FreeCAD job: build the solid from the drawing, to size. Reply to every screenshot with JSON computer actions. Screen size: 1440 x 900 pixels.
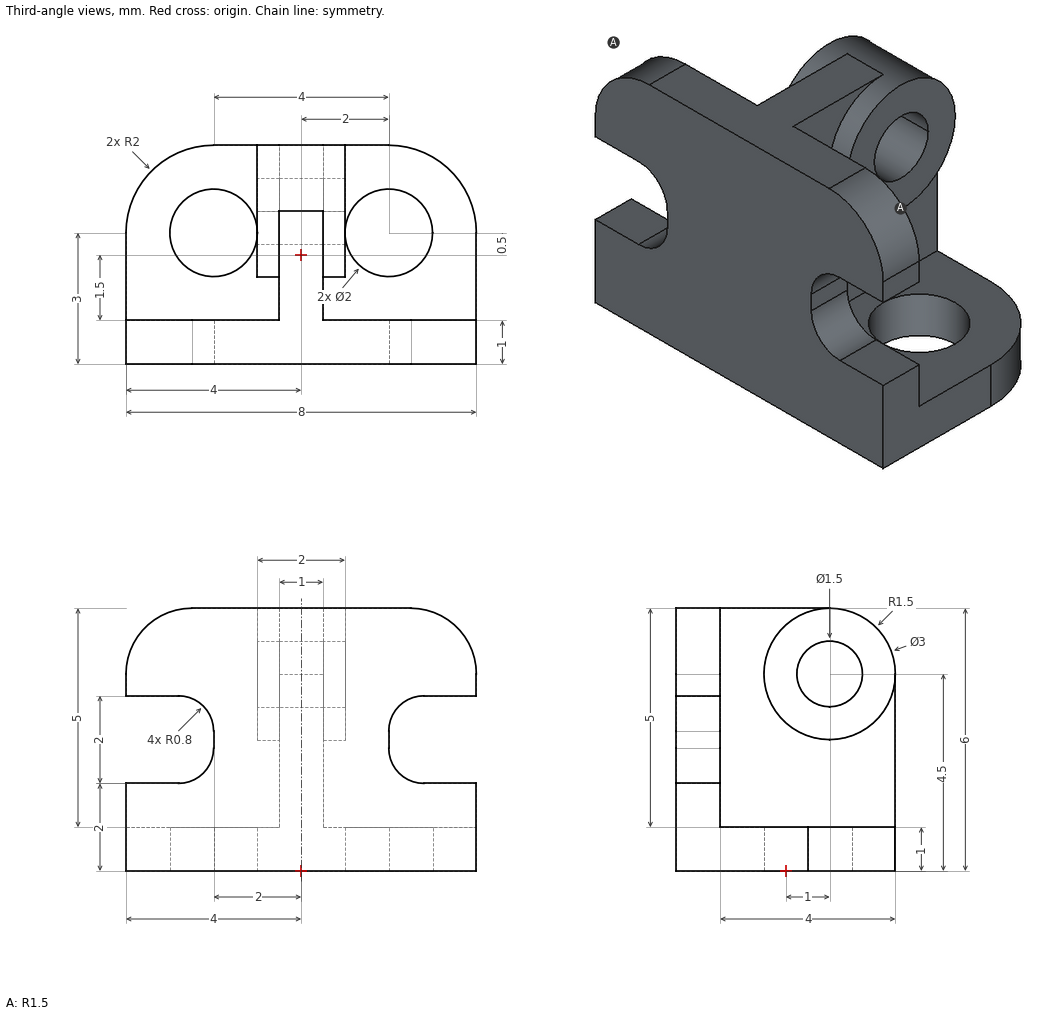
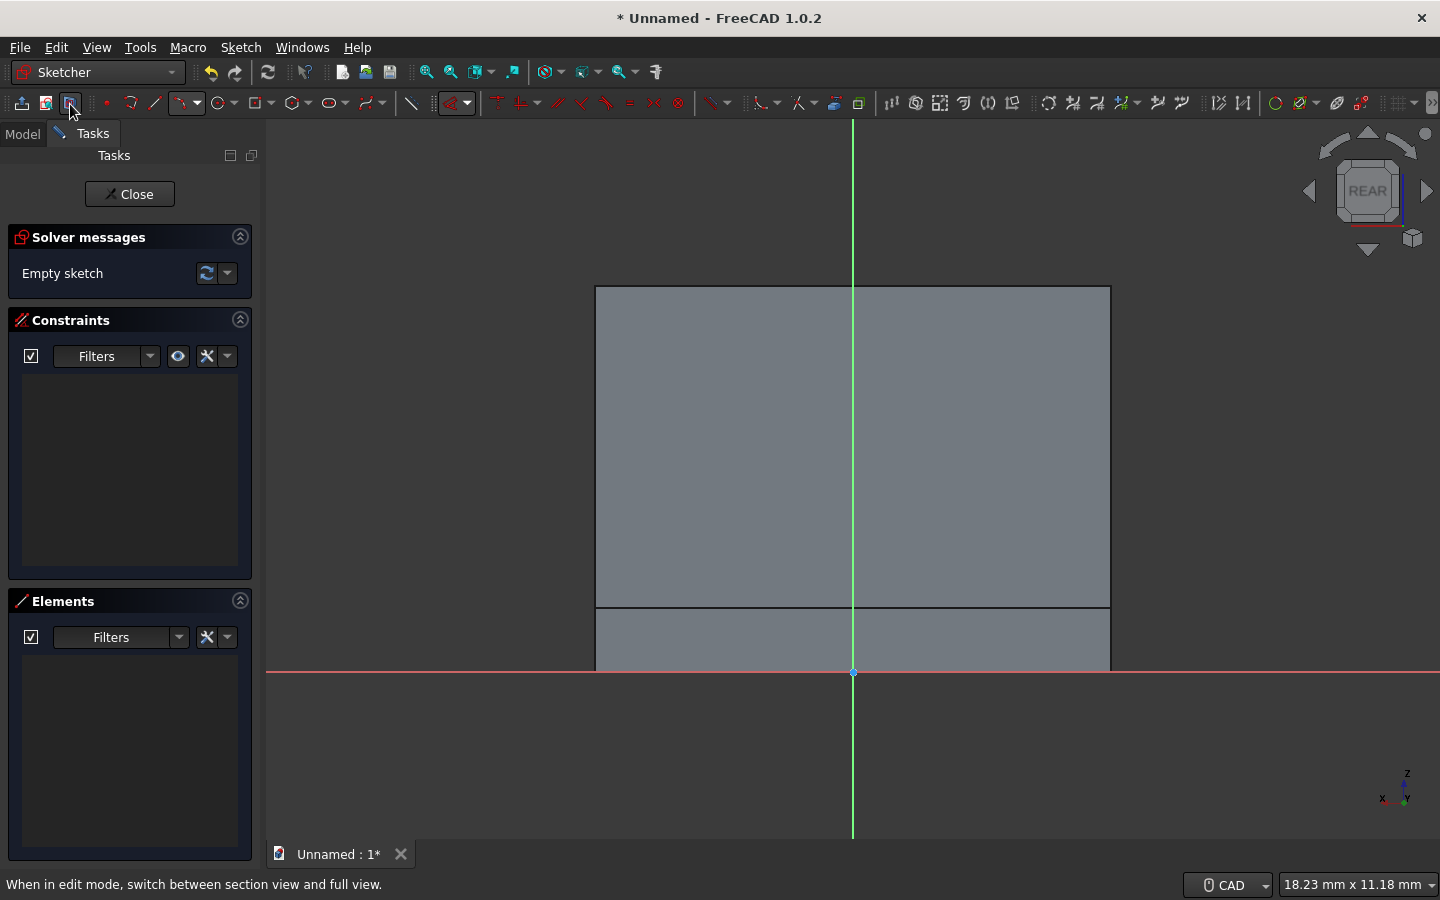
{"action": "left_click", "coordinate": [132, 104]}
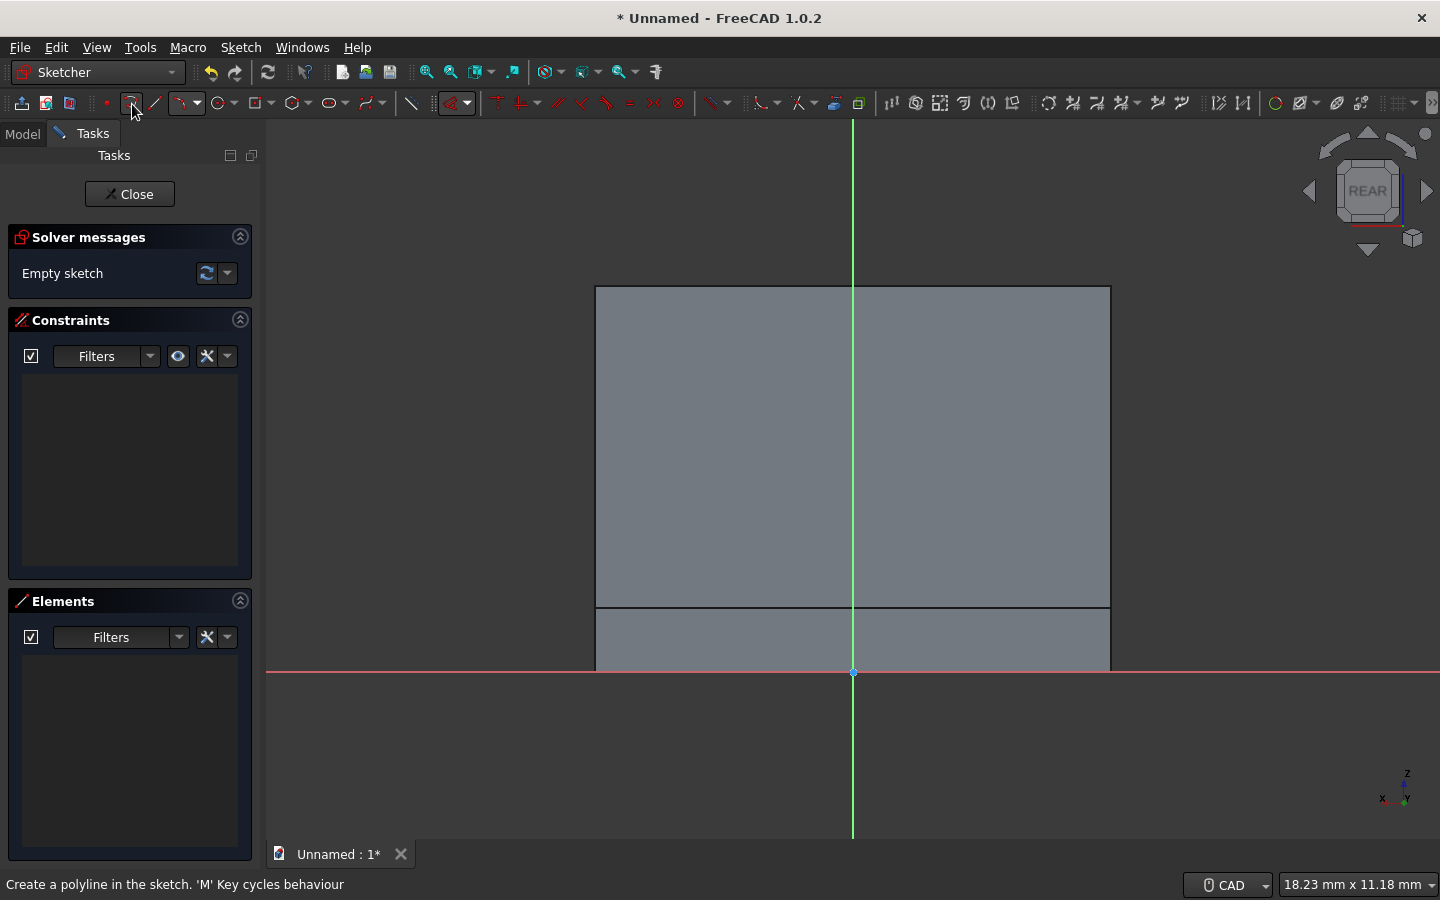
{"action": "left_click", "coordinate": [1033, 543]}
{"action": "left_click", "coordinate": [1111, 543]}
{"action": "left_click", "coordinate": [1111, 415]}
{"action": "left_click", "coordinate": [1033, 415]}
{"action": "right_click", "coordinate": [1033, 415]}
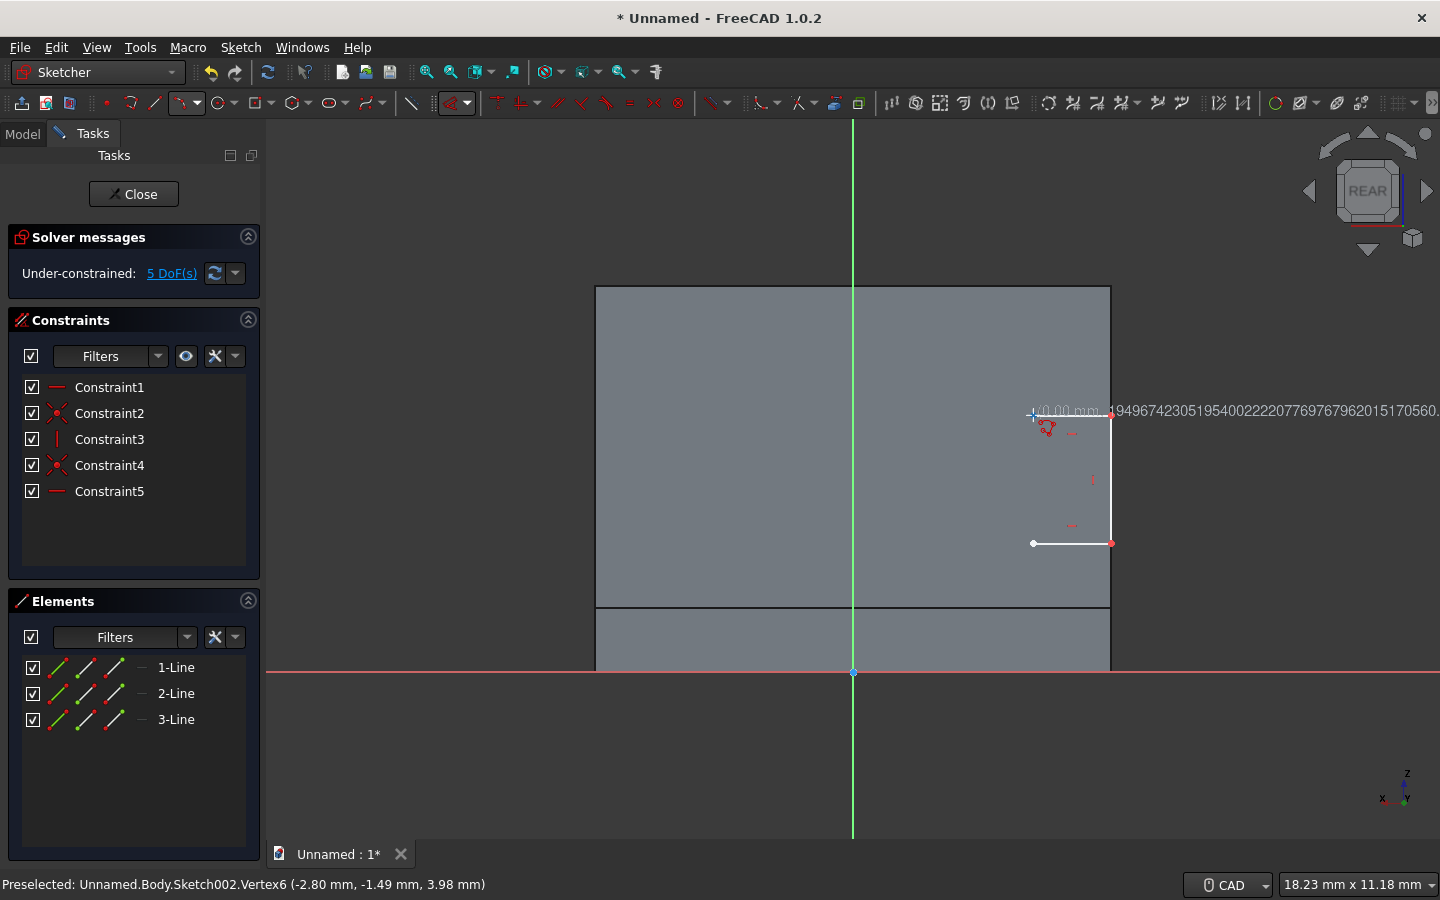
{"action": "left_click", "coordinate": [156, 104]}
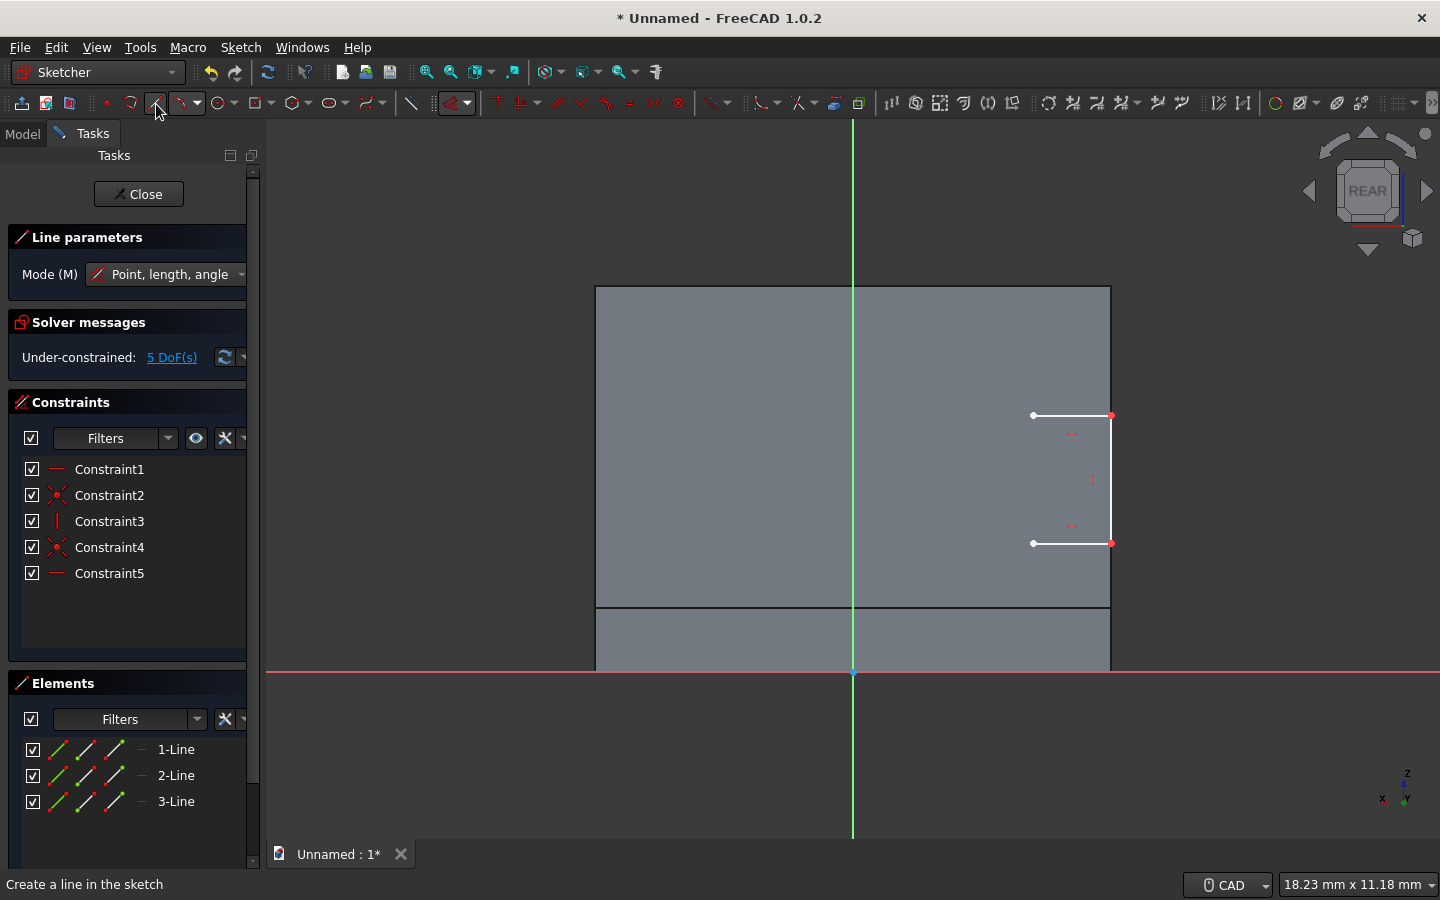
{"action": "left_click", "coordinate": [982, 466]}
{"action": "left_click", "coordinate": [982, 492]}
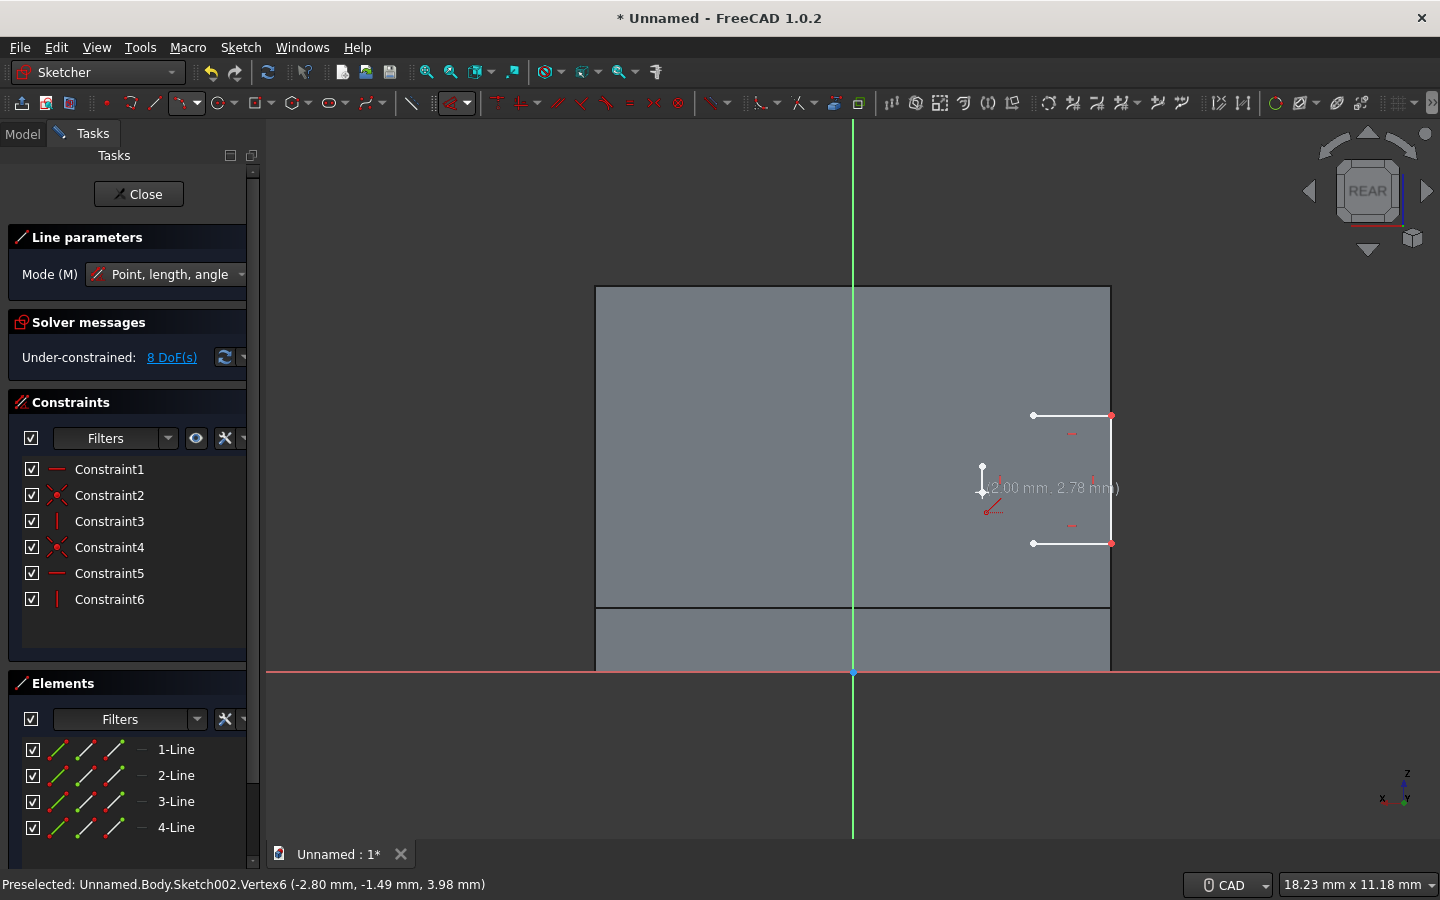
{"action": "left_click", "coordinate": [180, 104]}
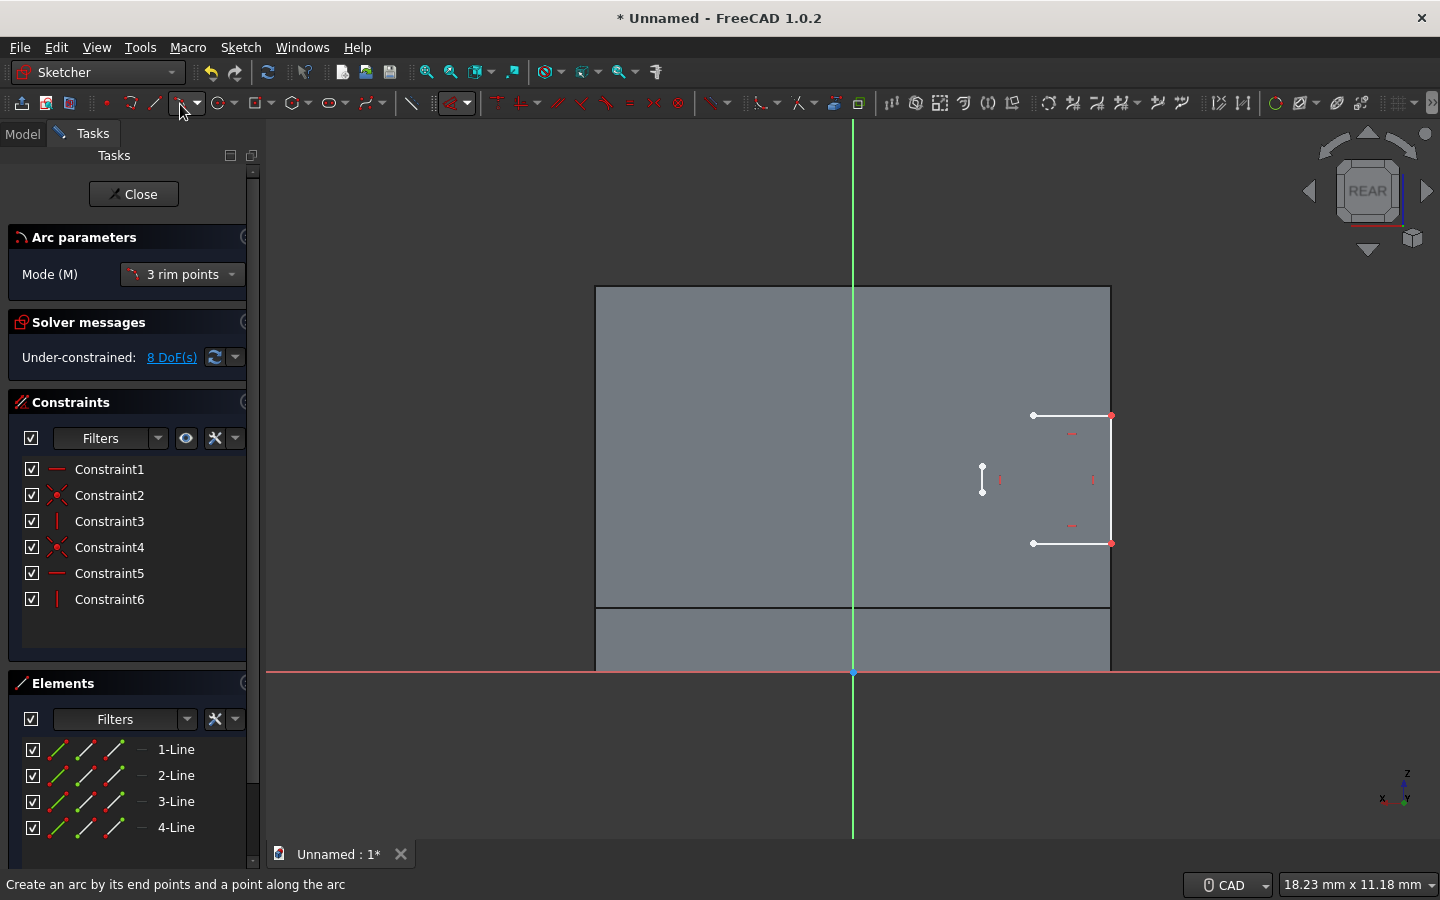
{"action": "left_click", "coordinate": [1033, 416]}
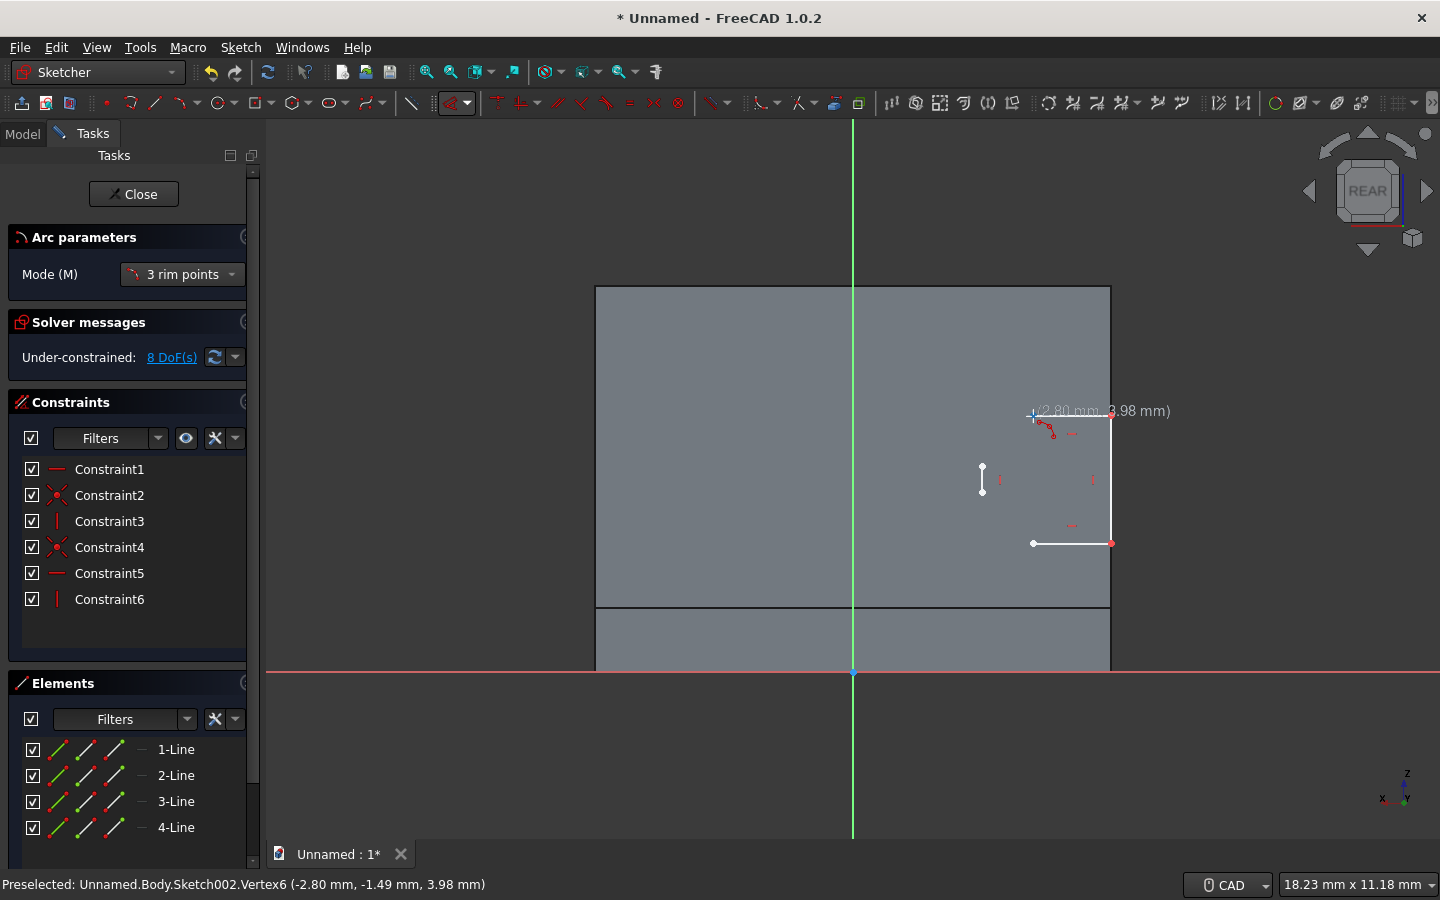
{"action": "scroll", "coordinate": [982, 466], "scroll_direction": "up", "scroll_amount": 2}